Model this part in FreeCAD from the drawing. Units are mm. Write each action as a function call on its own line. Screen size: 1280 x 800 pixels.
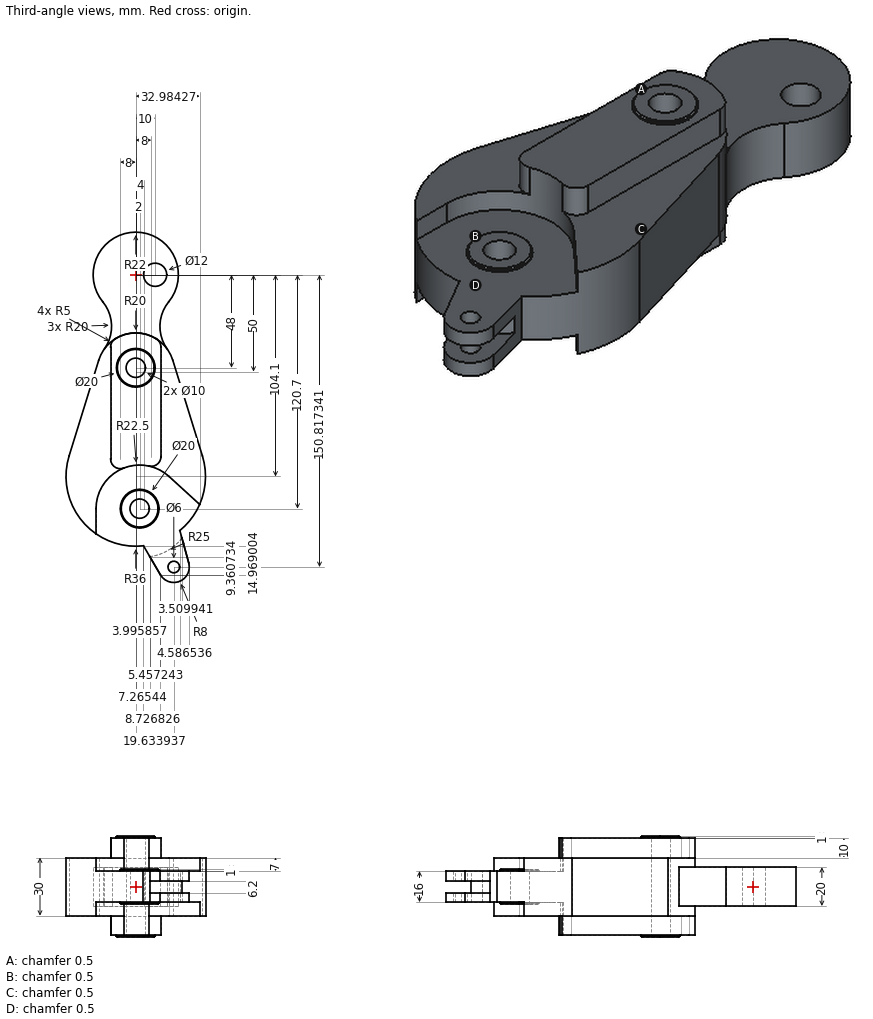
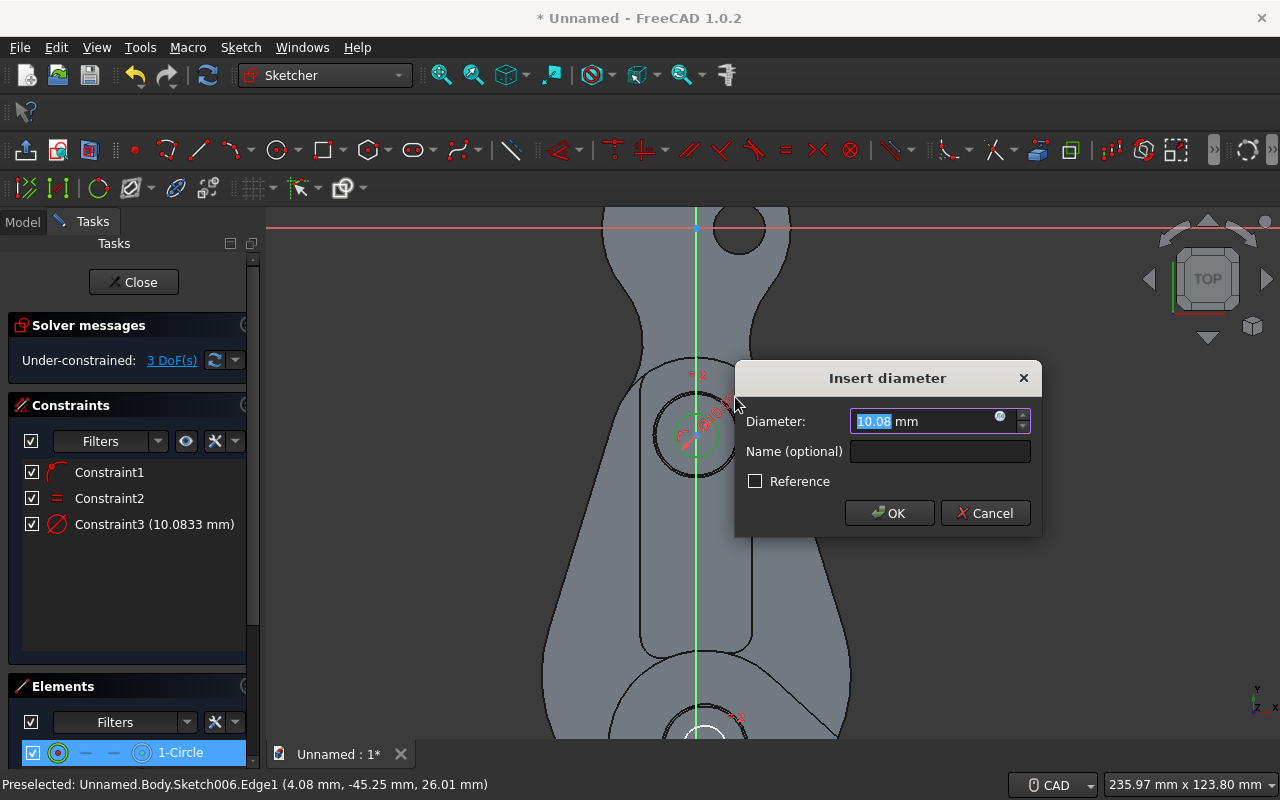
text(10)
key(Return)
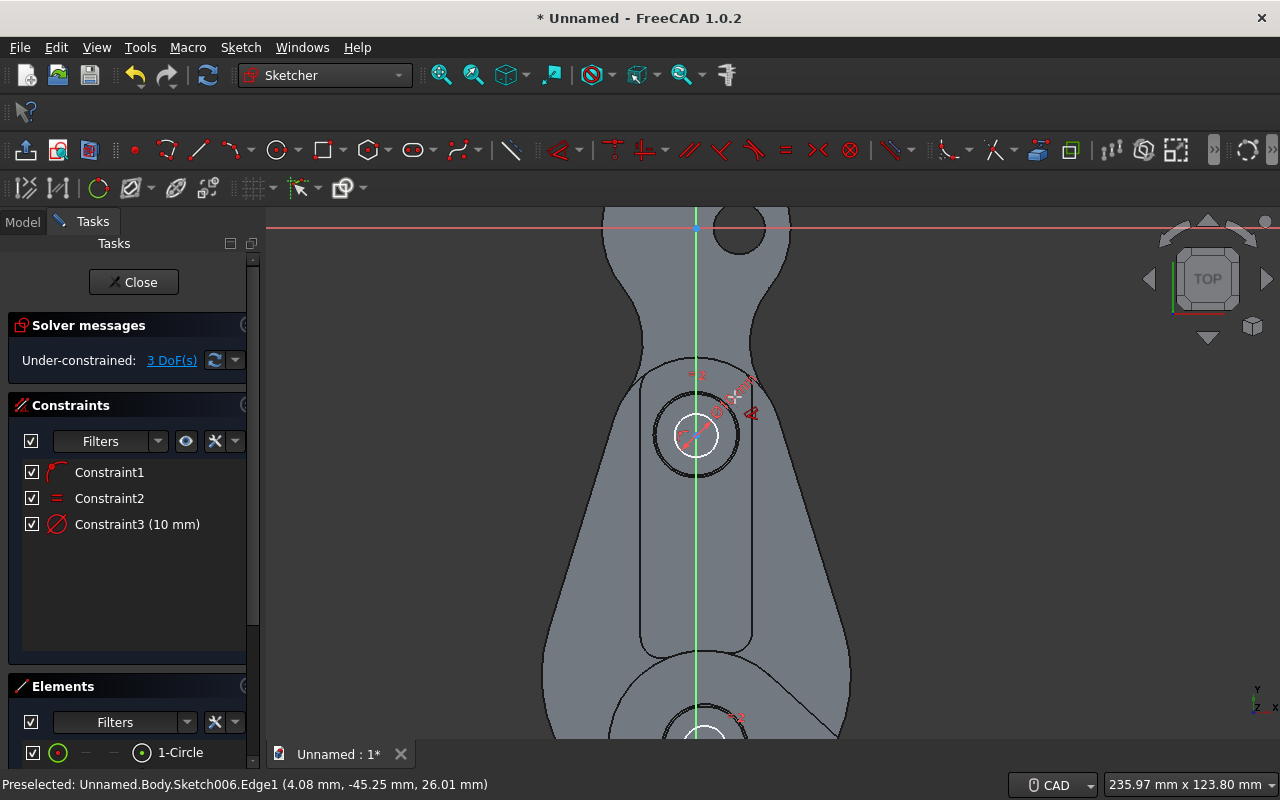
scroll(712, 421, down, 2)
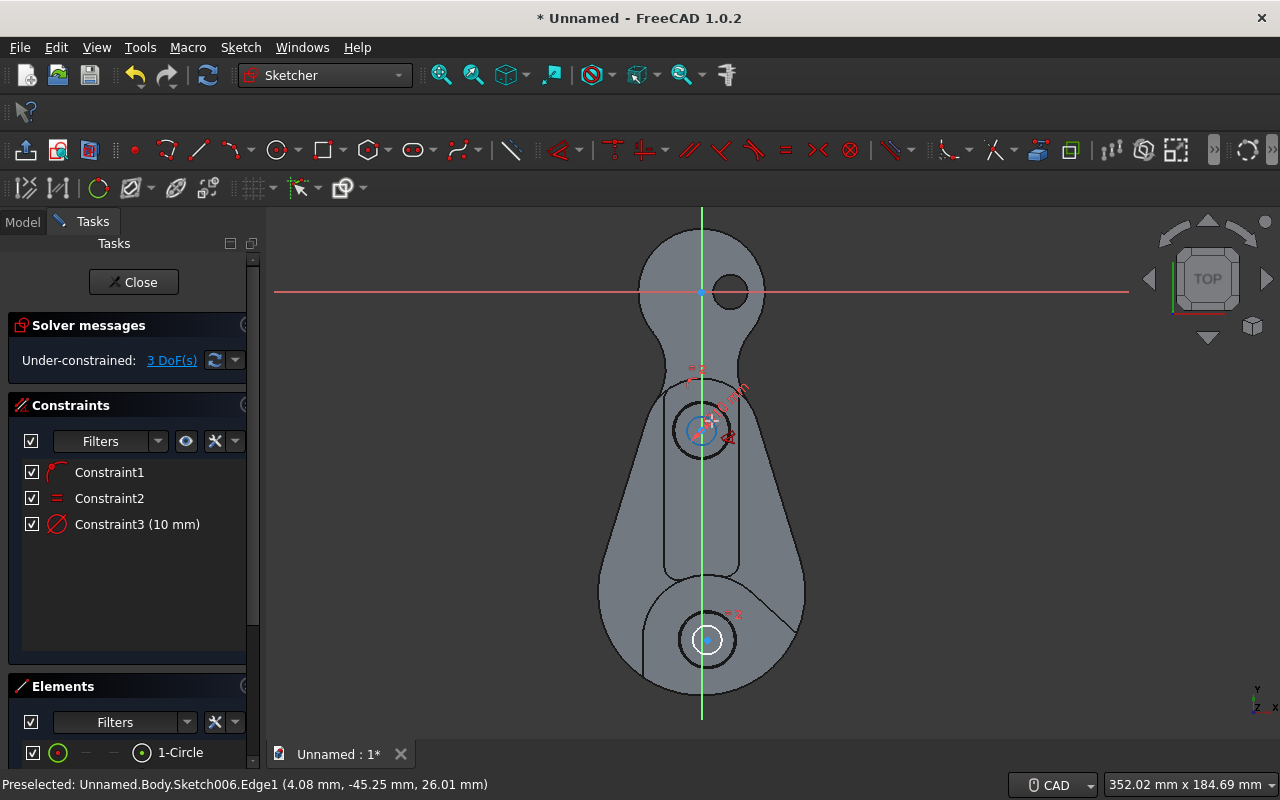
scroll(707, 640, up, 10)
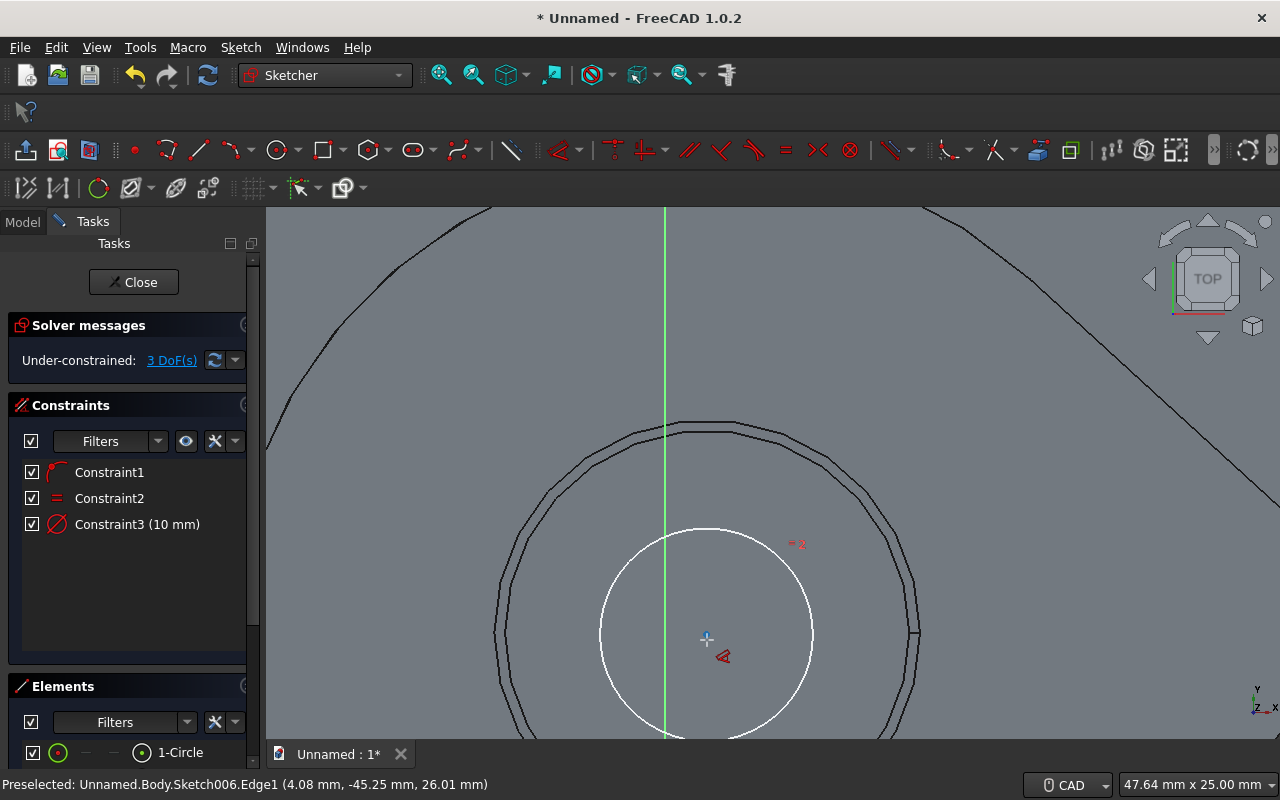
click(706, 635)
click(686, 669)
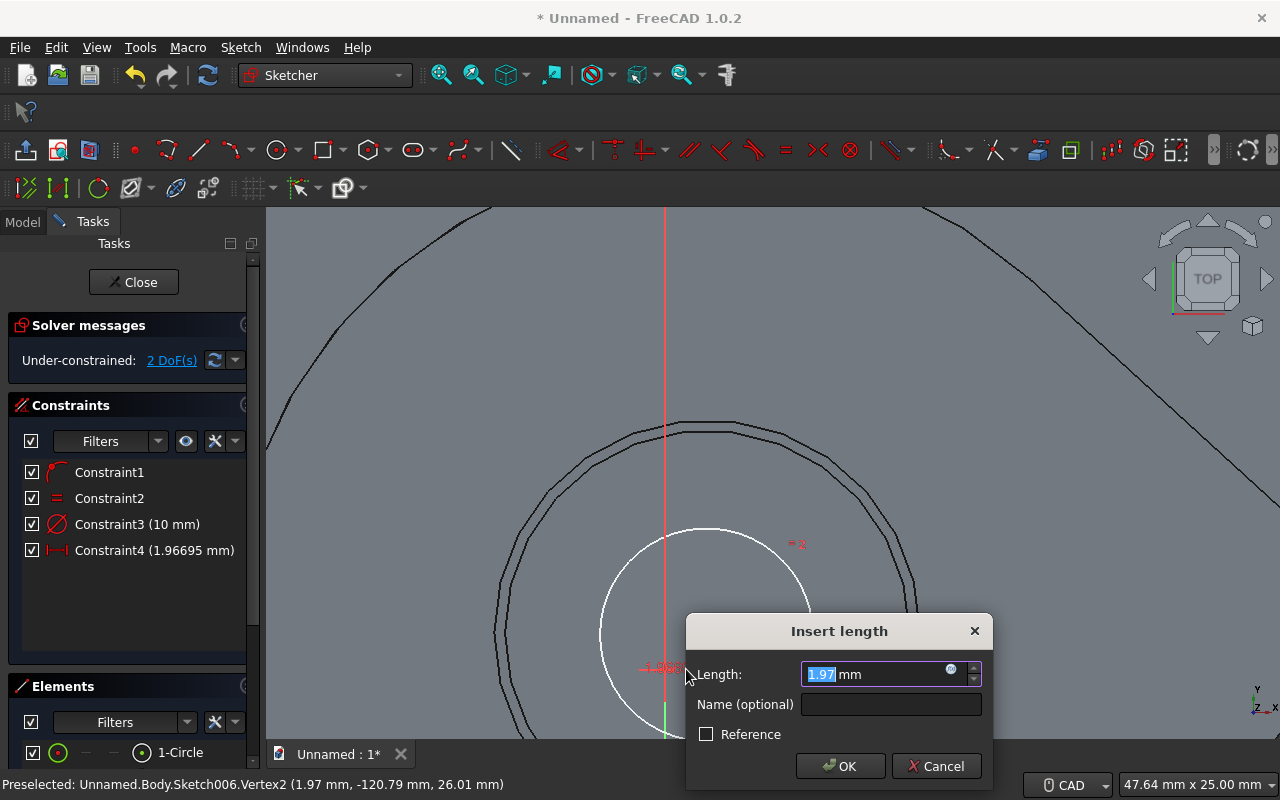
text(2)
key(Return)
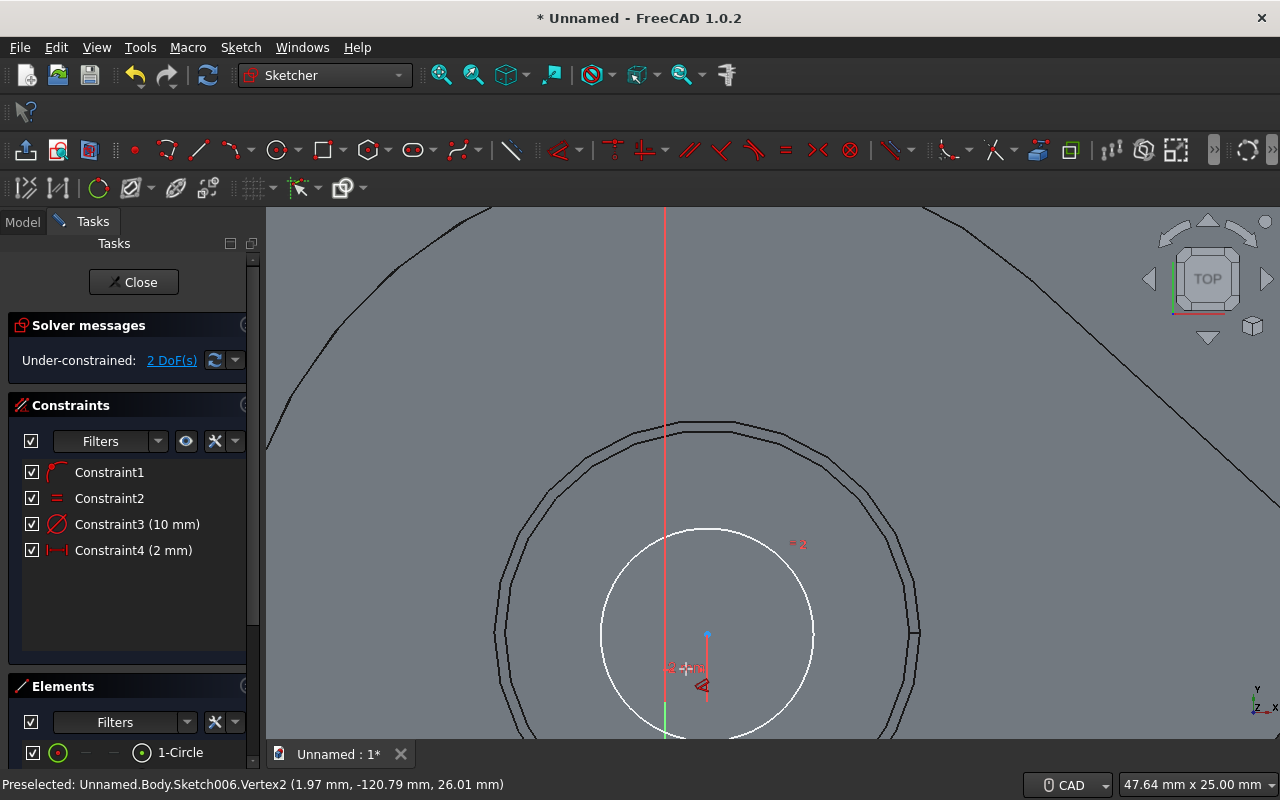
scroll(707, 641, down, 10)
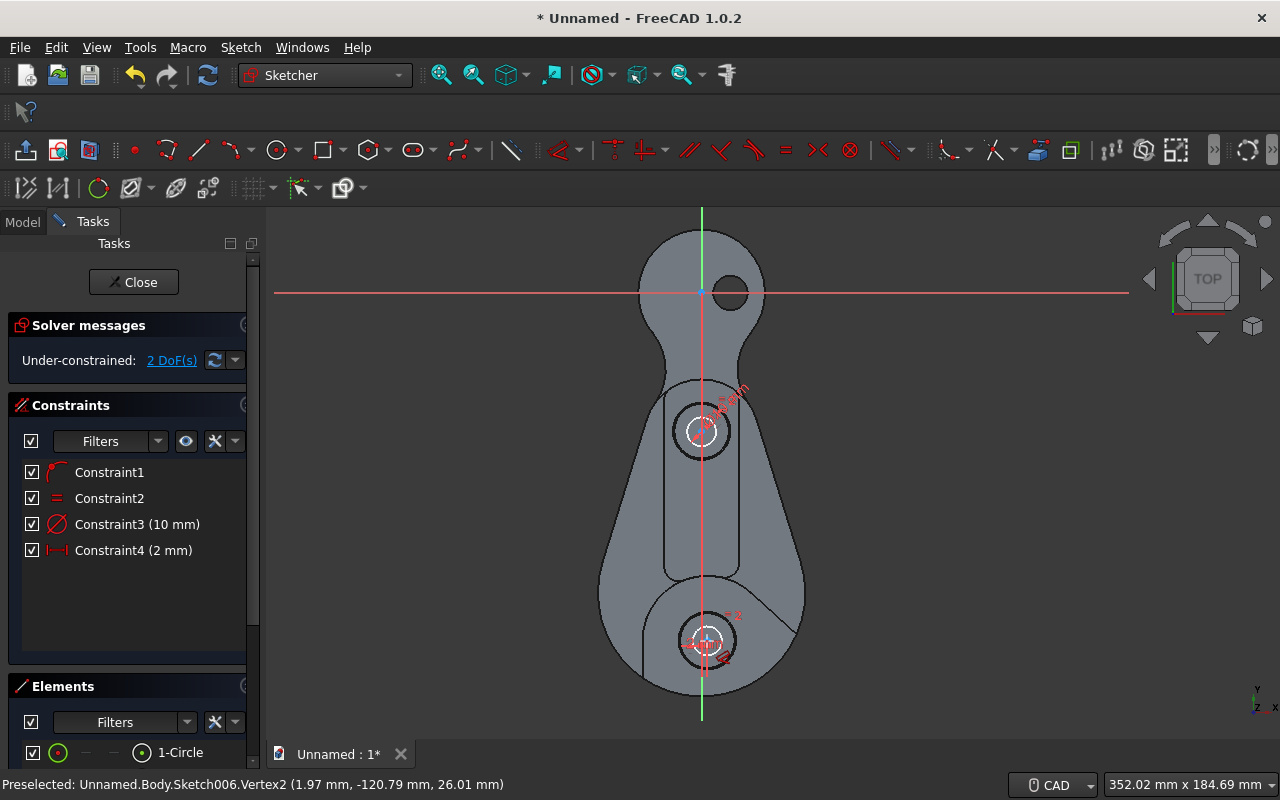
click(702, 432)
click(668, 362)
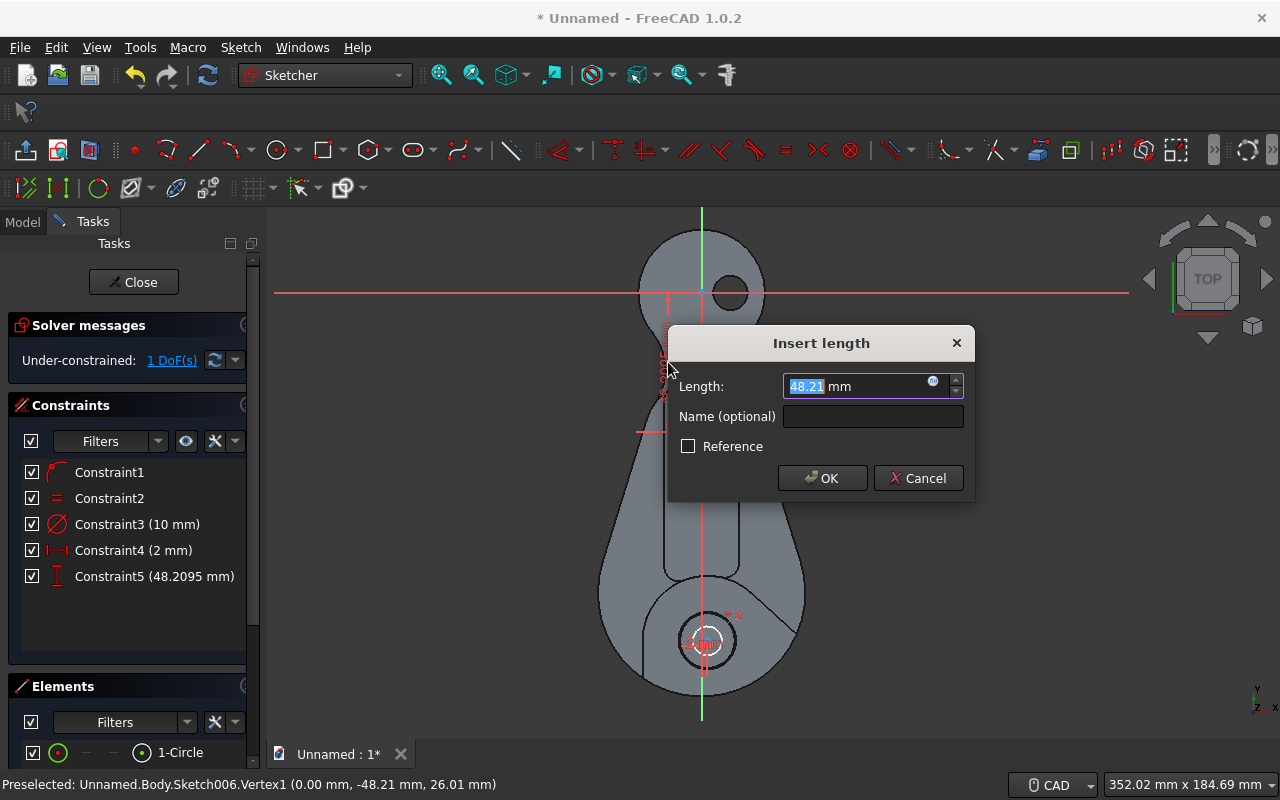
text(48)
key(Return)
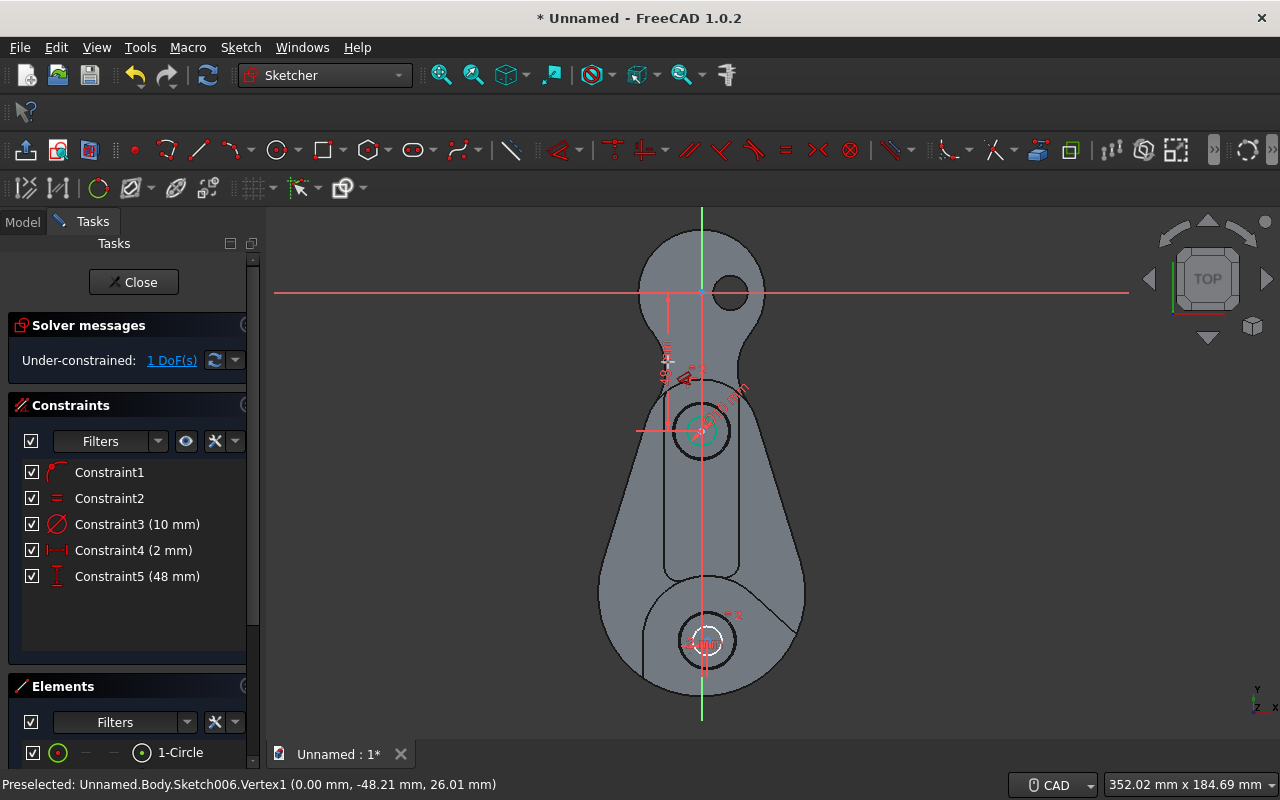
click(707, 641)
click(741, 467)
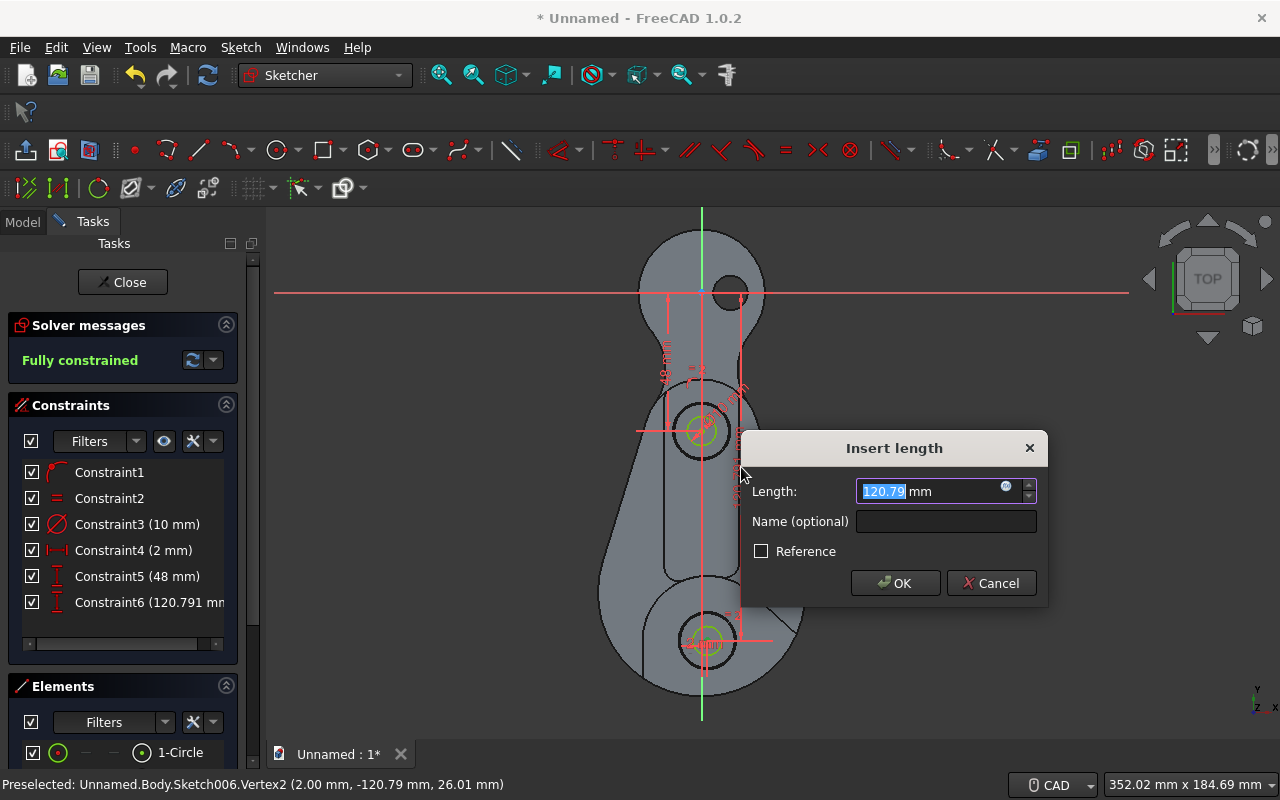
text(120.7)
key(Return)
key(Escape)